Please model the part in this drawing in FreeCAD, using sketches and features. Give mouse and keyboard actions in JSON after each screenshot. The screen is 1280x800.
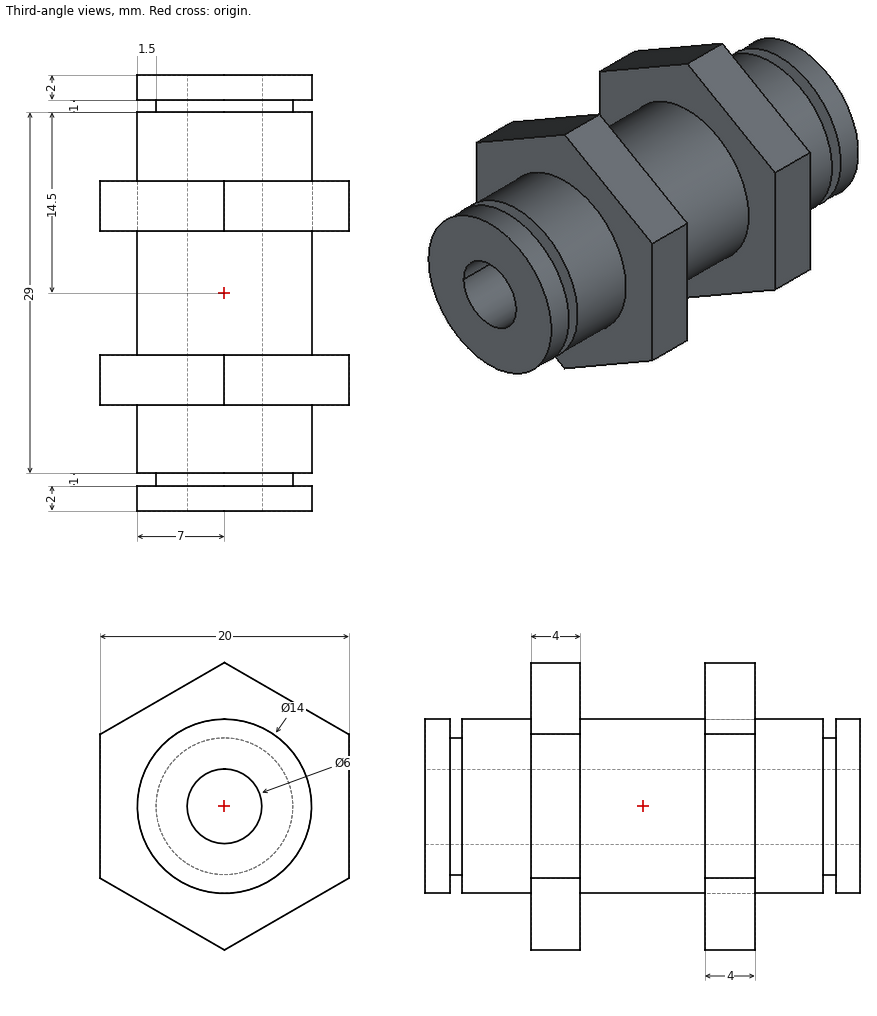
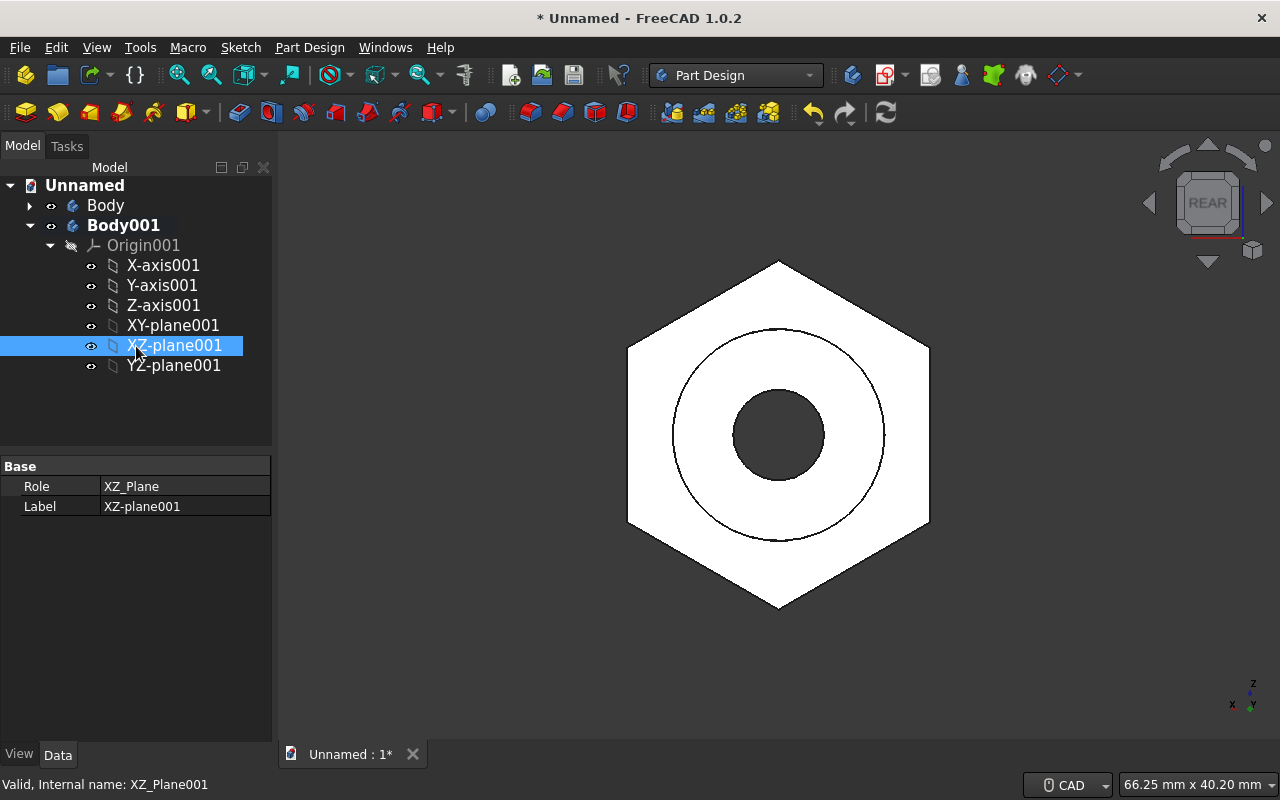
{"action": "left_click", "coordinate": [1058, 76]}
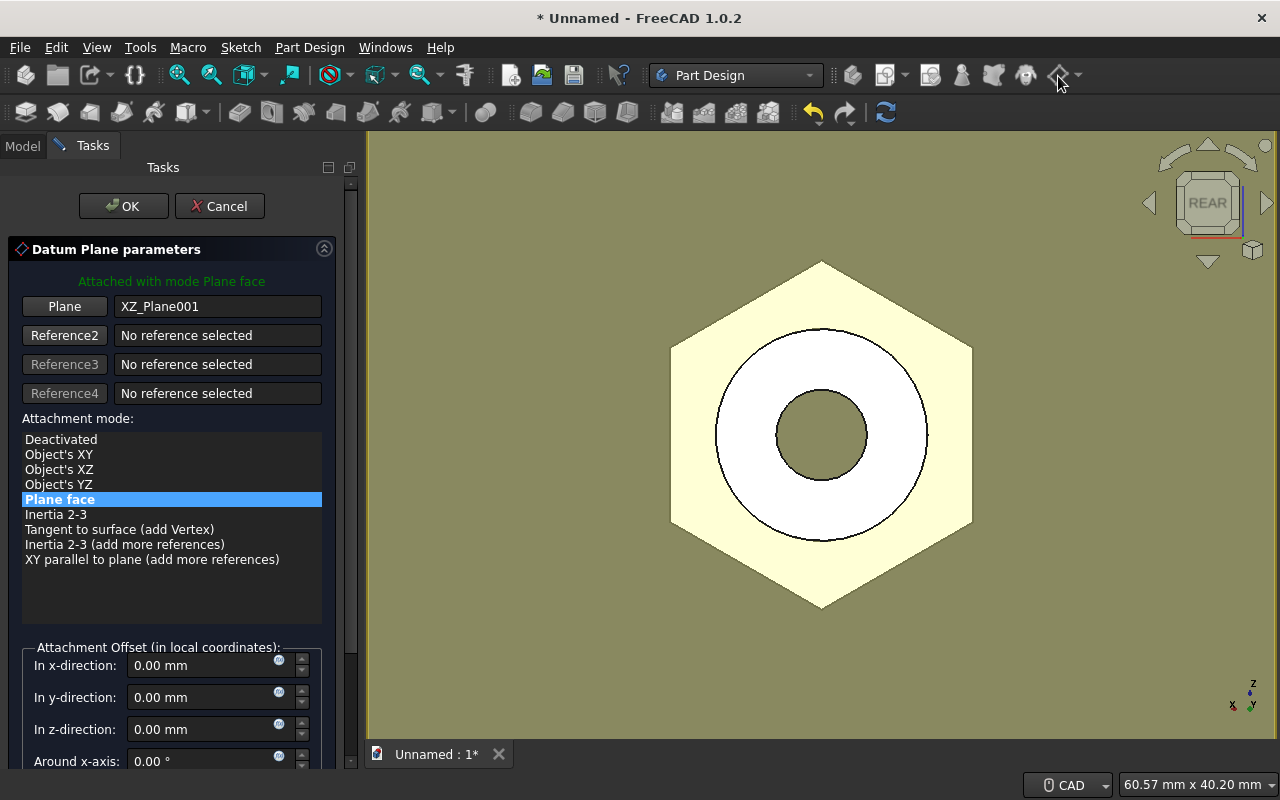
{"action": "triple_click", "coordinate": [210, 729]}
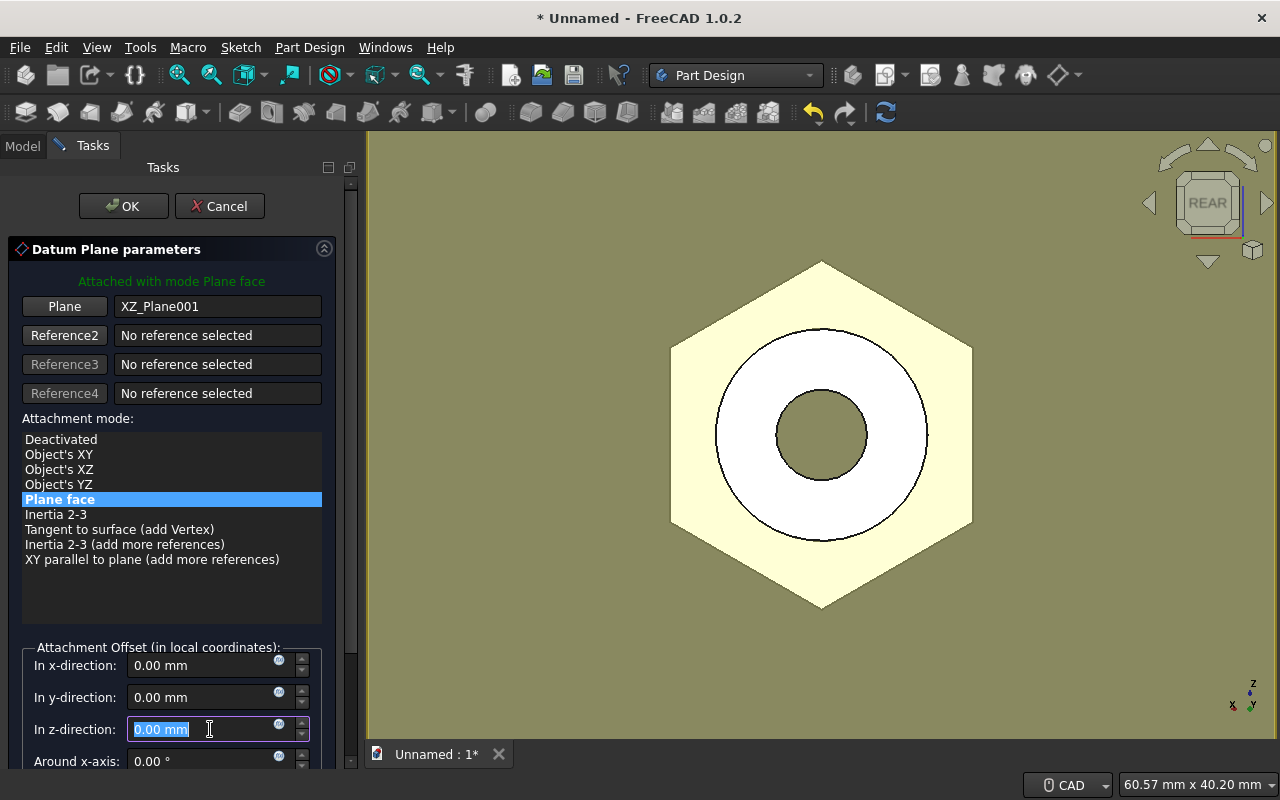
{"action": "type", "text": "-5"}
{"action": "key", "text": "Tab"}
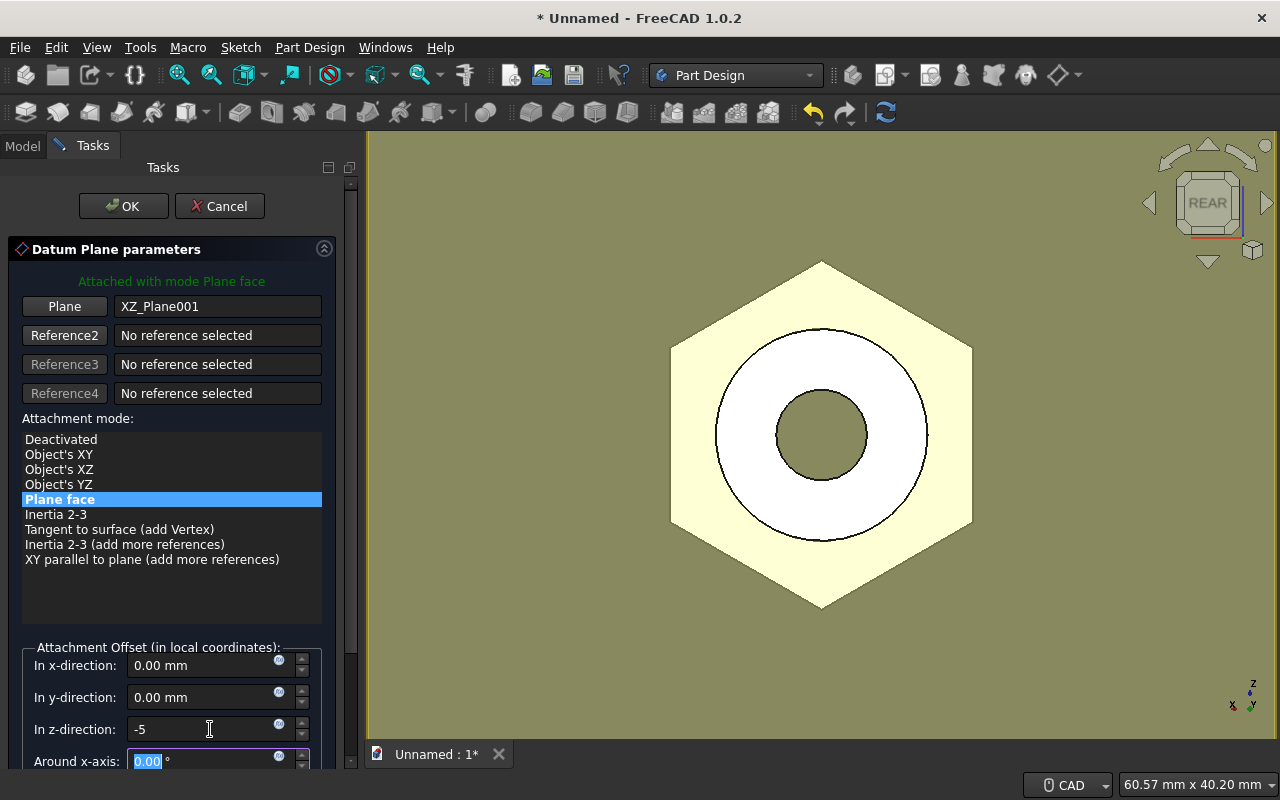
{"action": "left_click", "coordinate": [124, 206]}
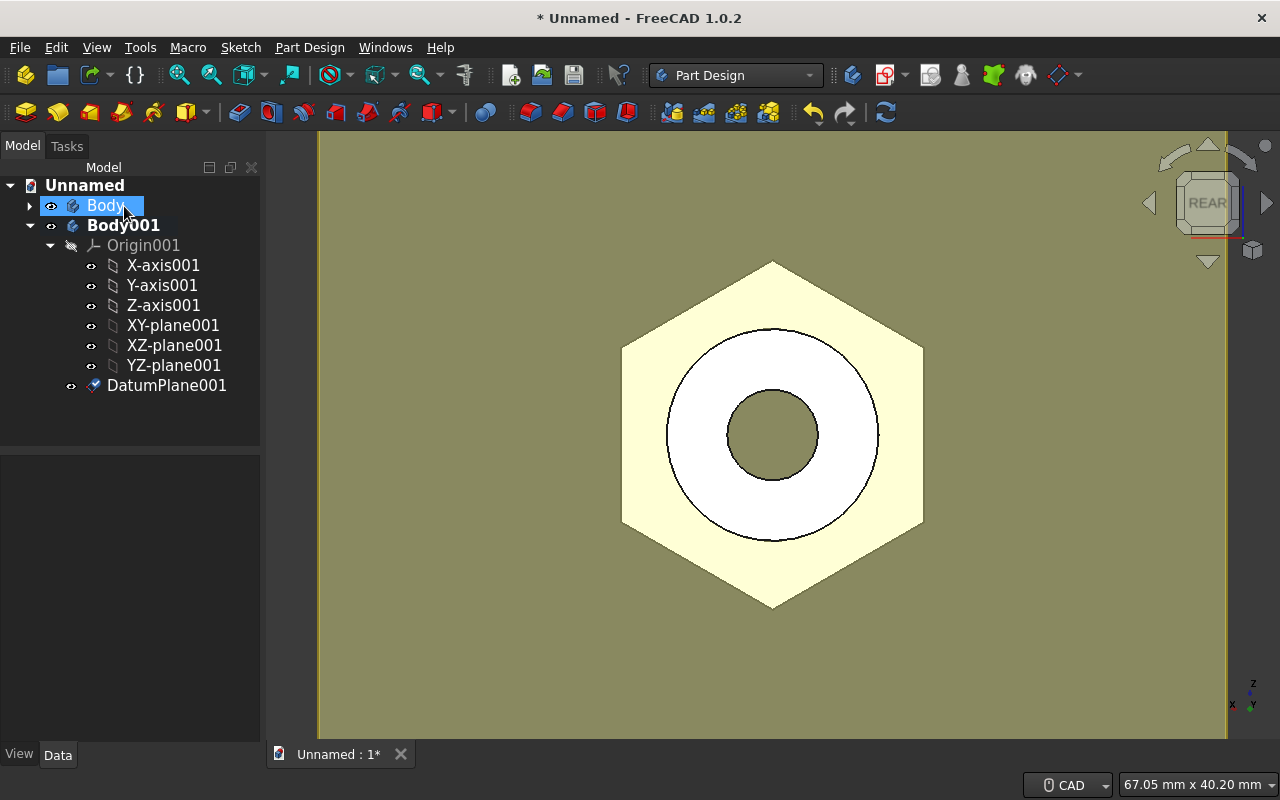
{"action": "left_click", "coordinate": [116, 386]}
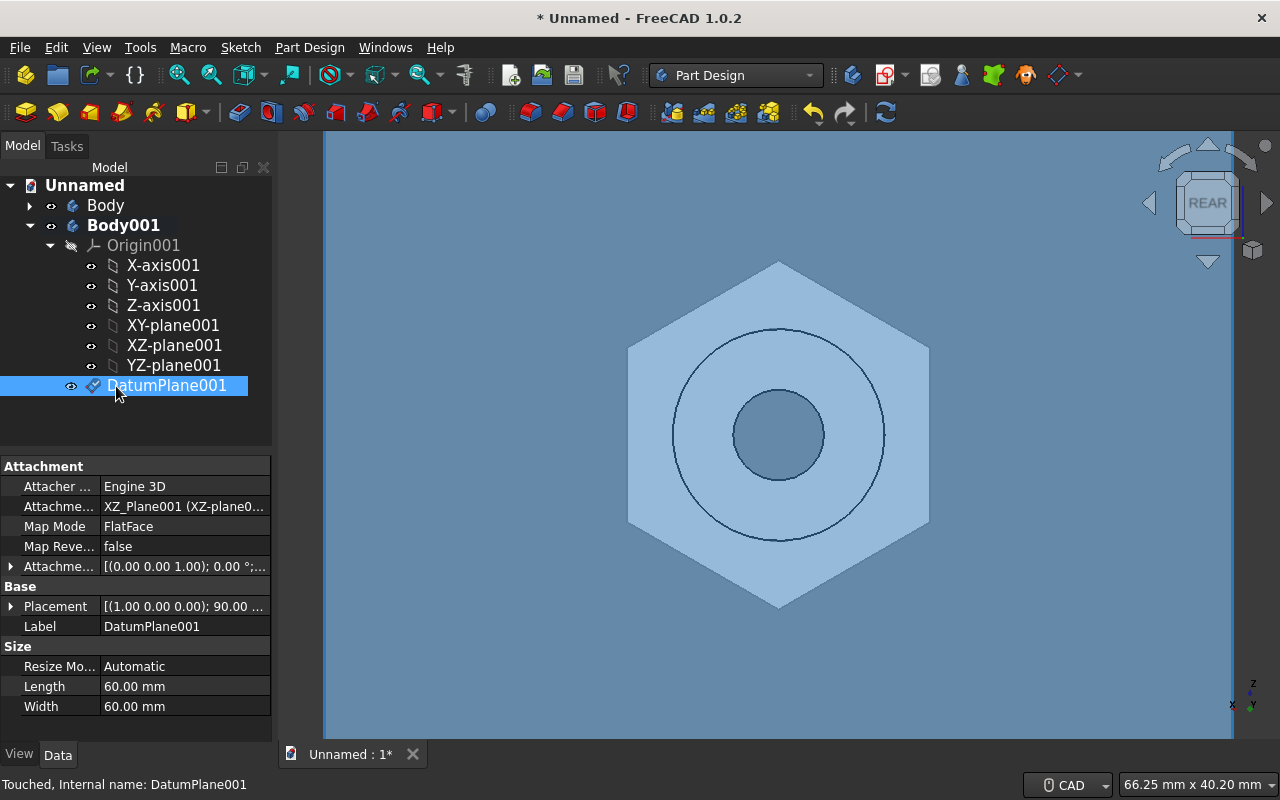
{"action": "left_click", "coordinate": [886, 76]}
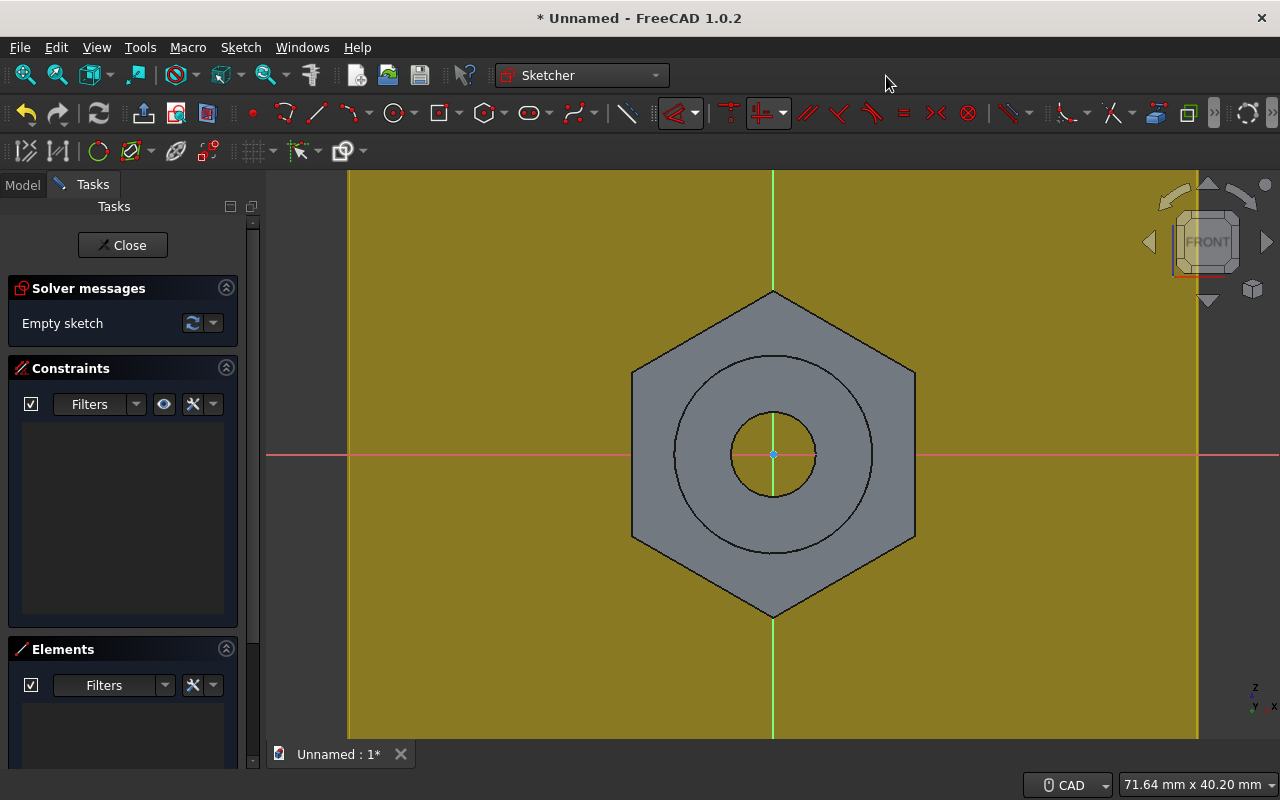
{"action": "left_click", "coordinate": [484, 114]}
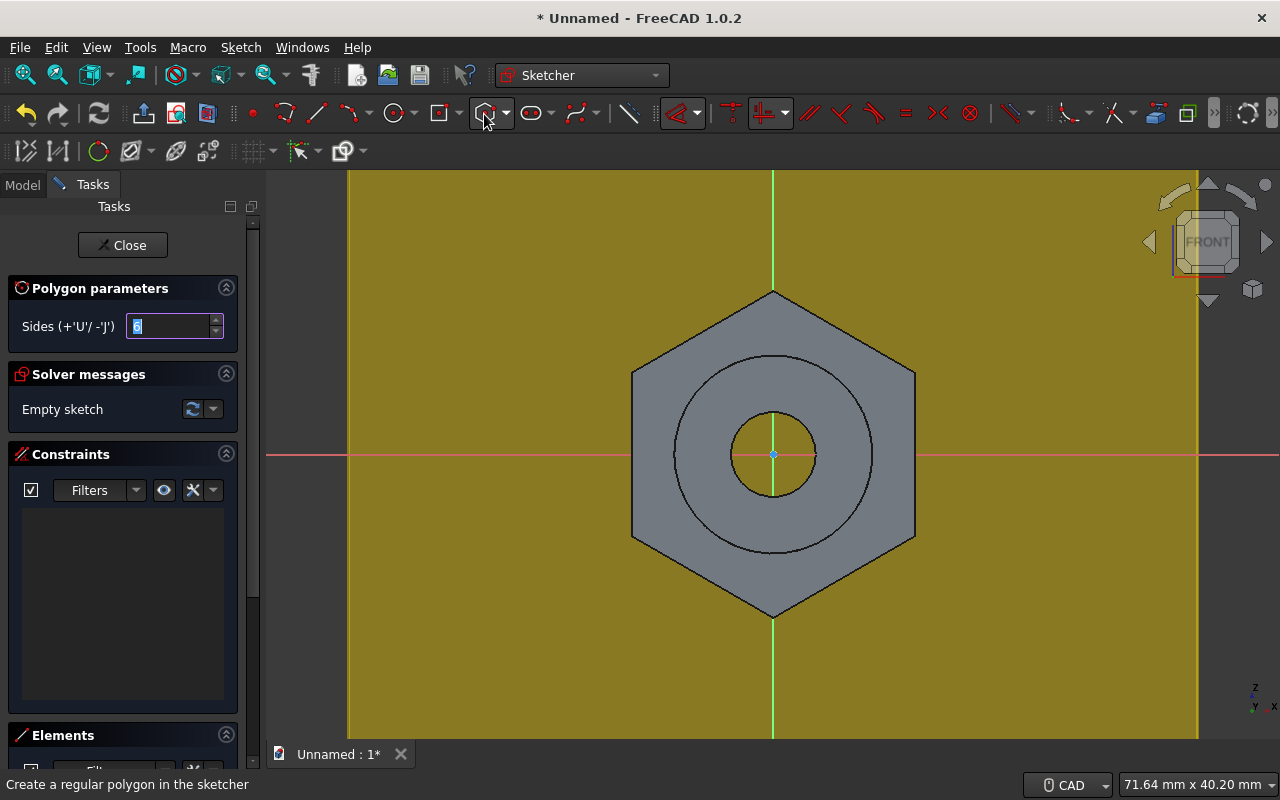
{"action": "left_click", "coordinate": [773, 455]}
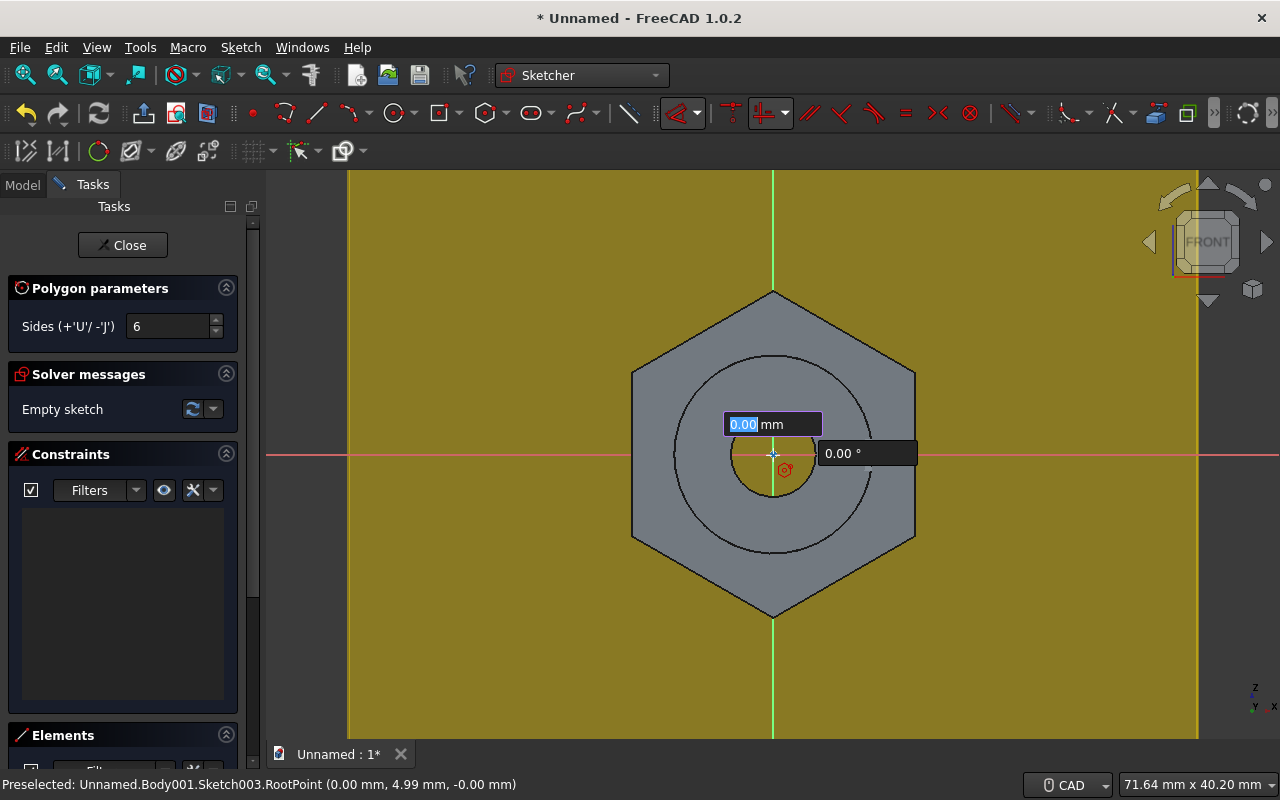
{"action": "left_click", "coordinate": [773, 618]}
{"action": "key", "text": "Escape"}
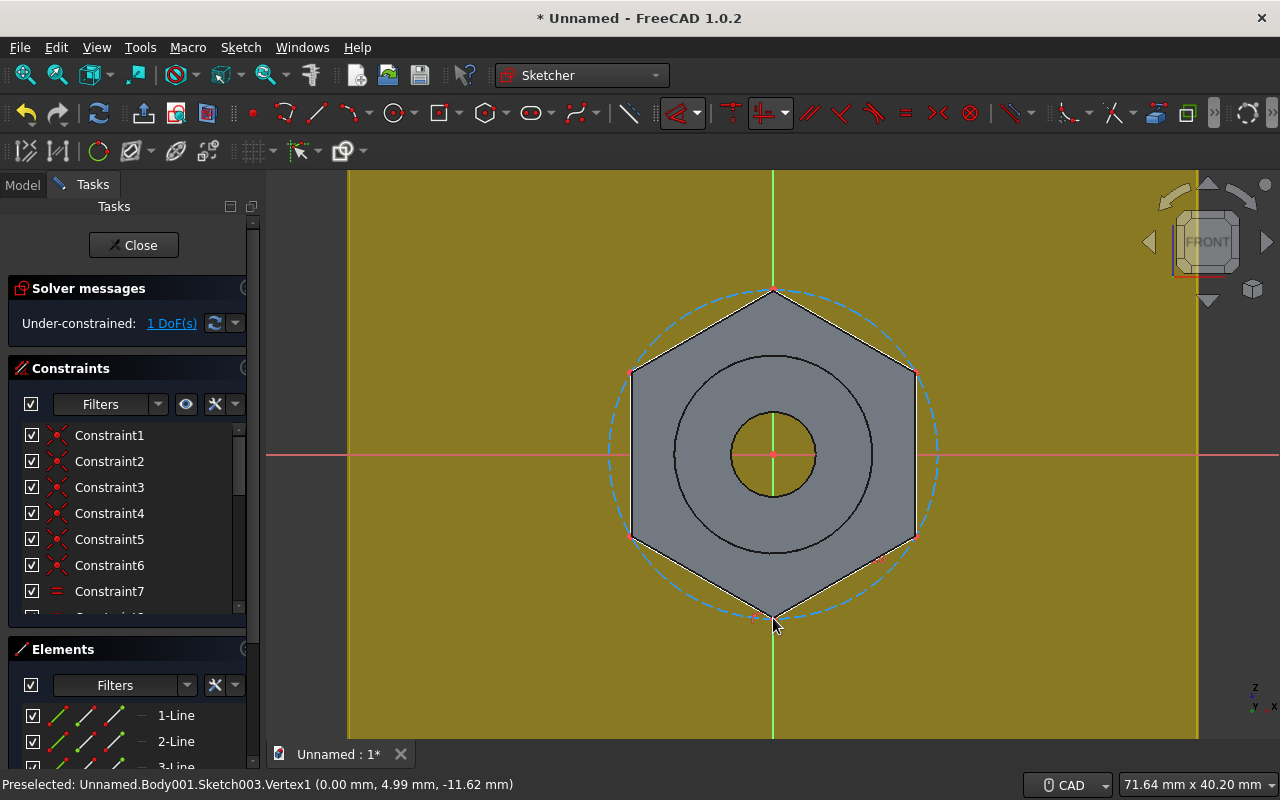
{"action": "left_click", "coordinate": [394, 114]}